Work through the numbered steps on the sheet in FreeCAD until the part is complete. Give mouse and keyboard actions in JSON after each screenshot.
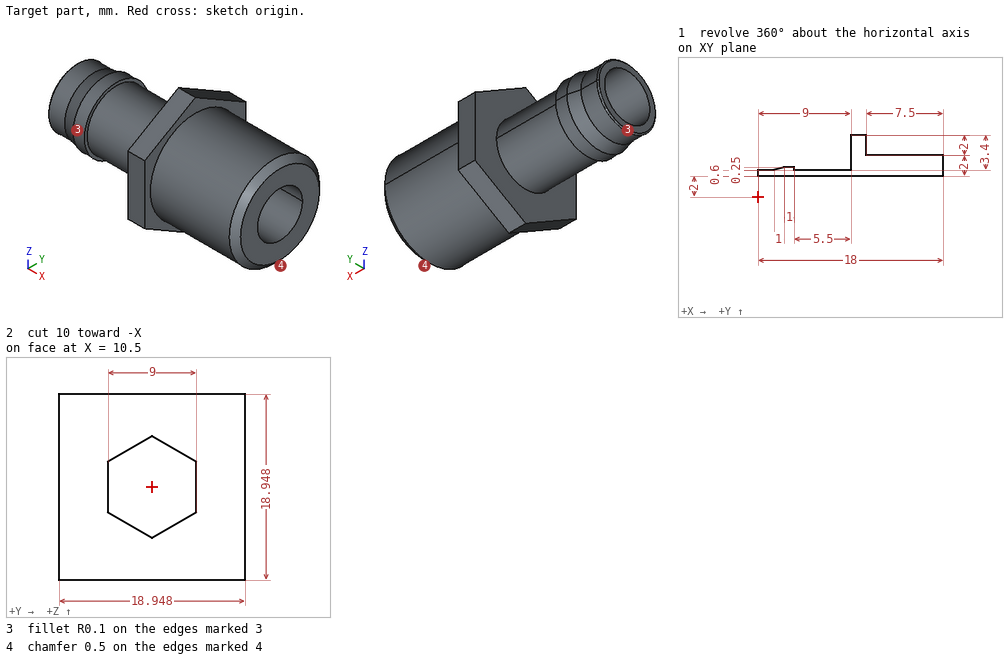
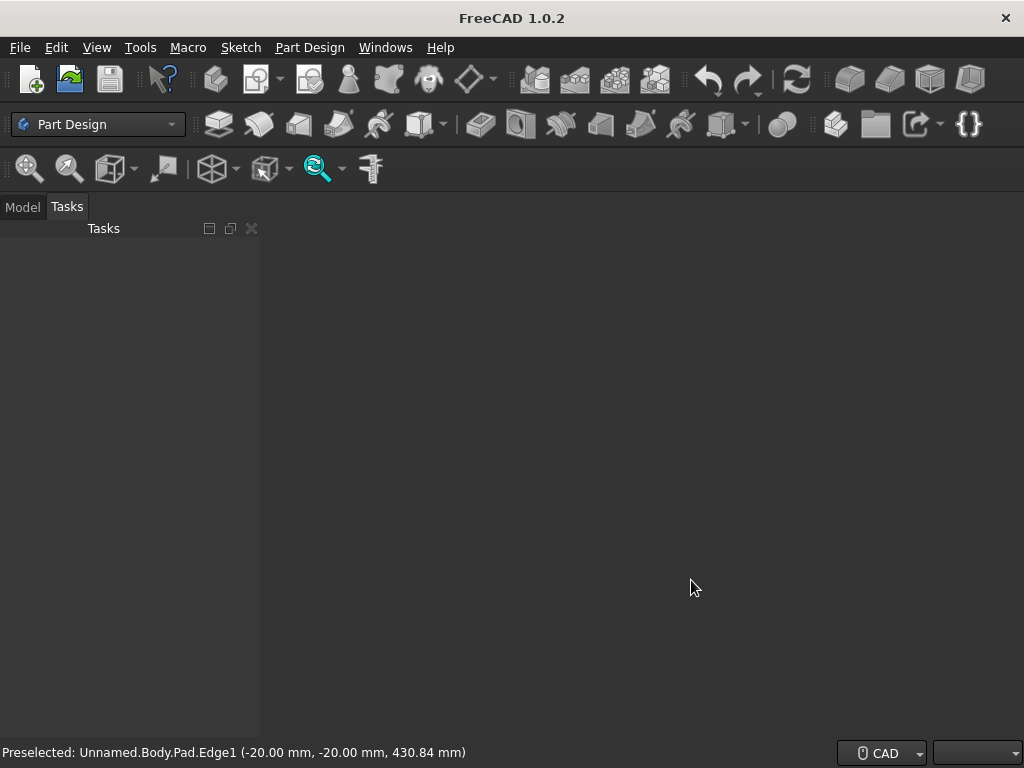
{"action": "left_click", "coordinate": [30, 80]}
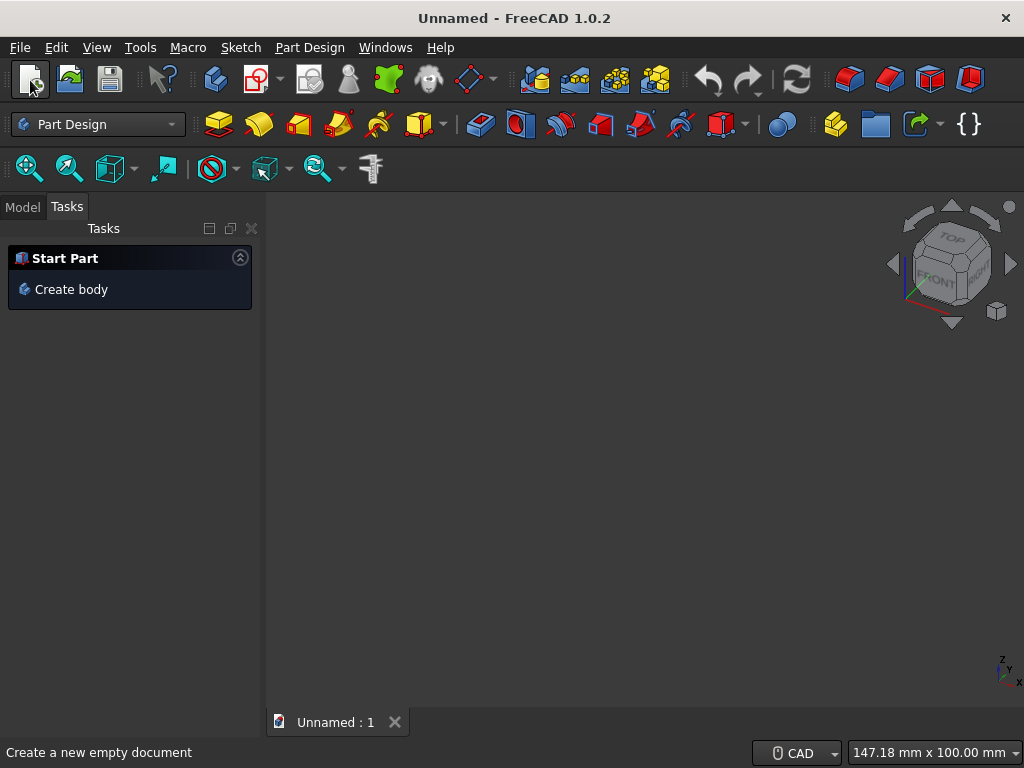
{"action": "left_click", "coordinate": [256, 80]}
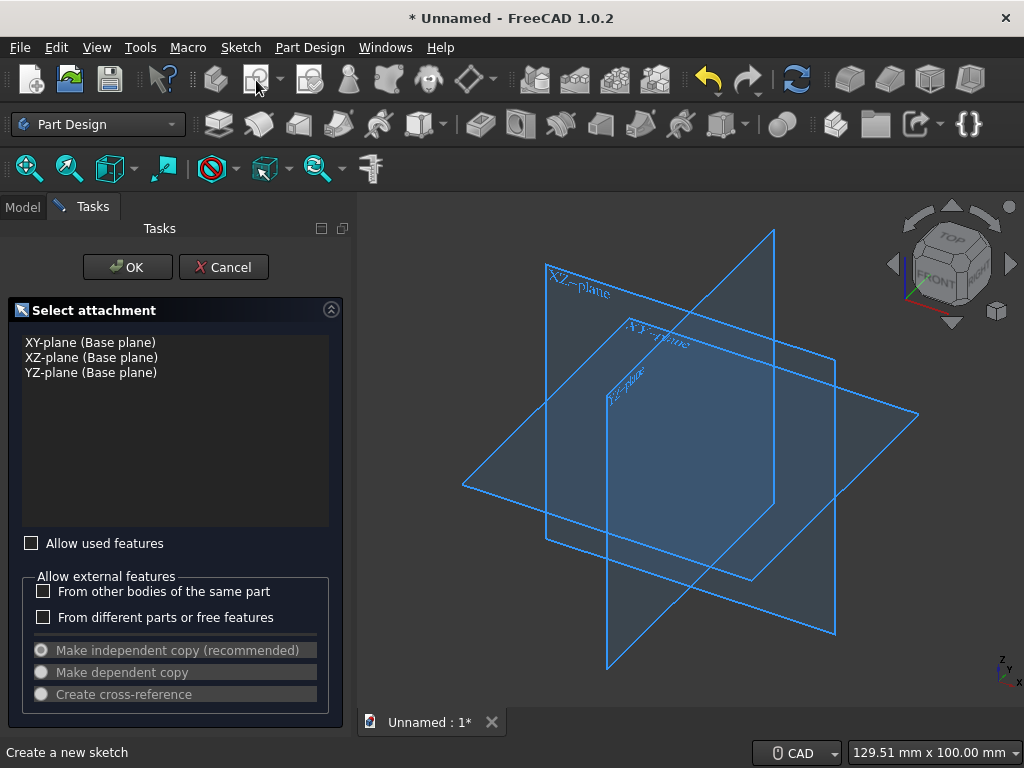
{"action": "left_click", "coordinate": [82, 342]}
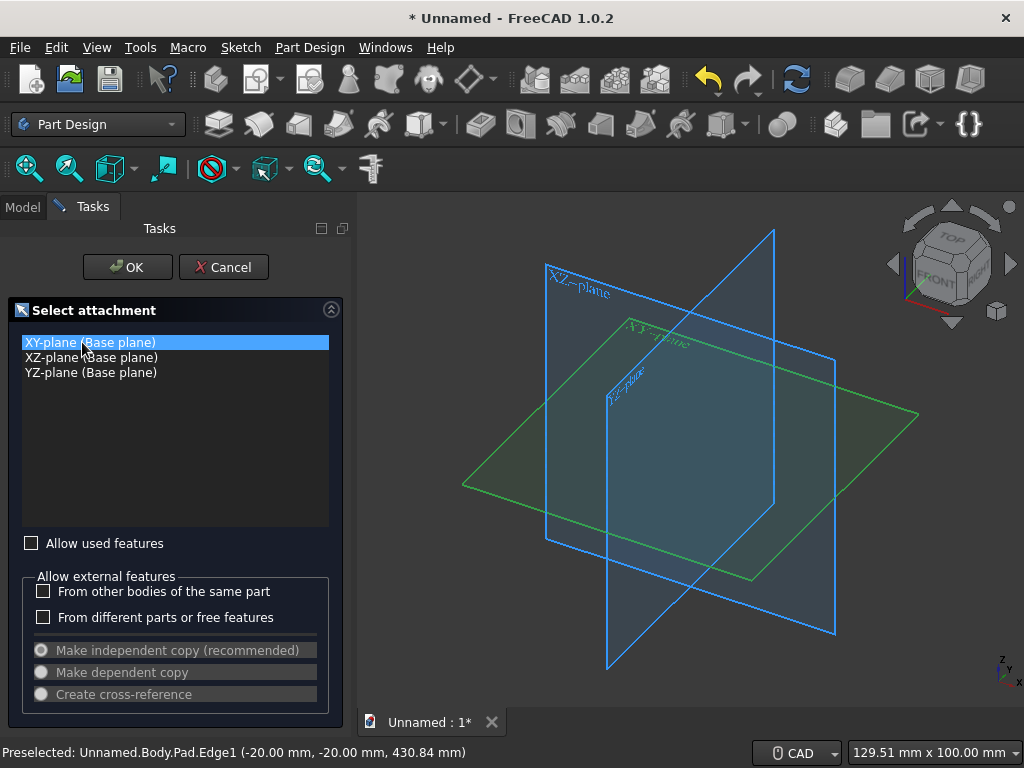
{"action": "left_click", "coordinate": [128, 267]}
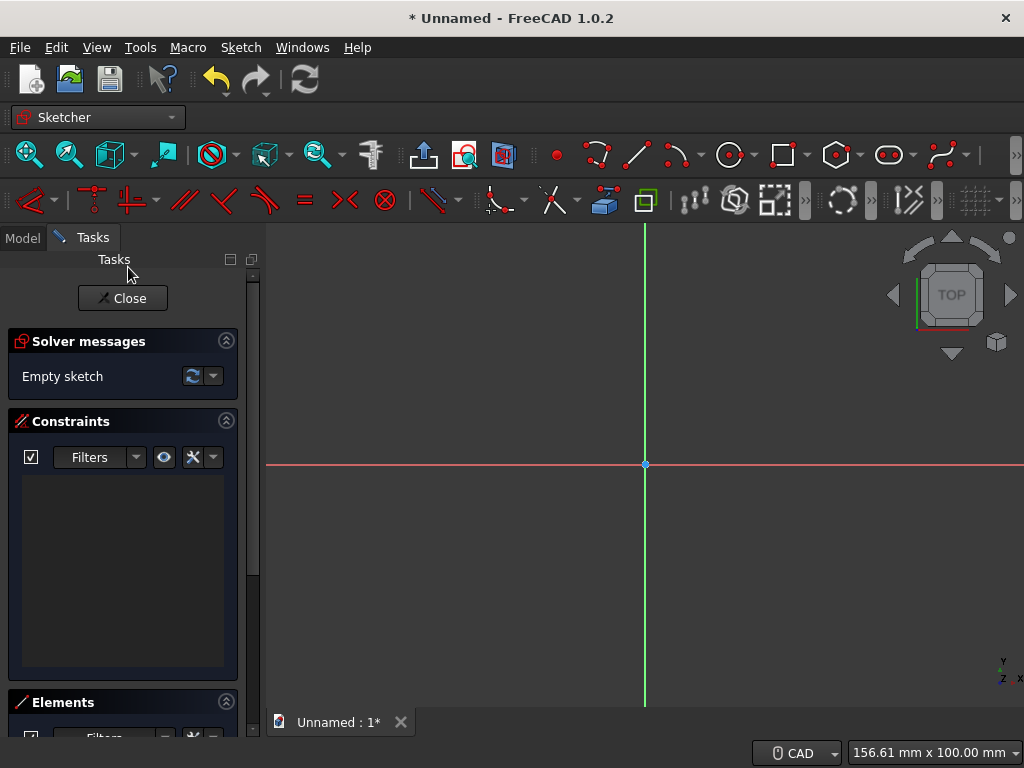
{"action": "scroll", "coordinate": [717, 447], "scroll_direction": "up", "scroll_amount": 8}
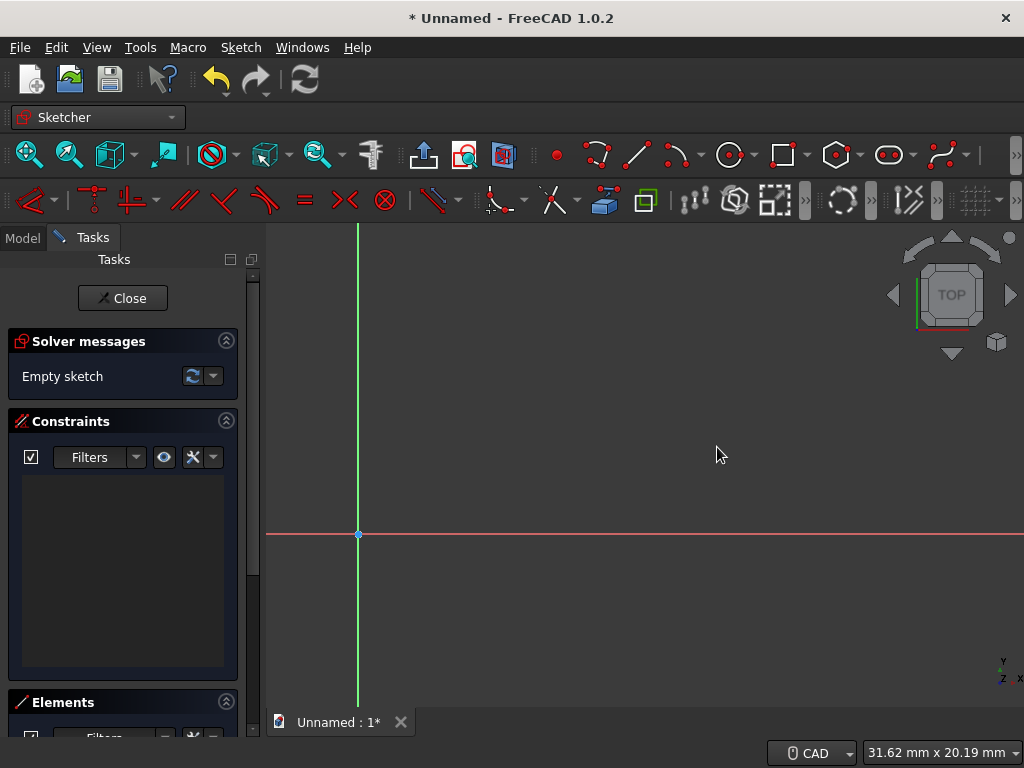
{"action": "left_click", "coordinate": [598, 156]}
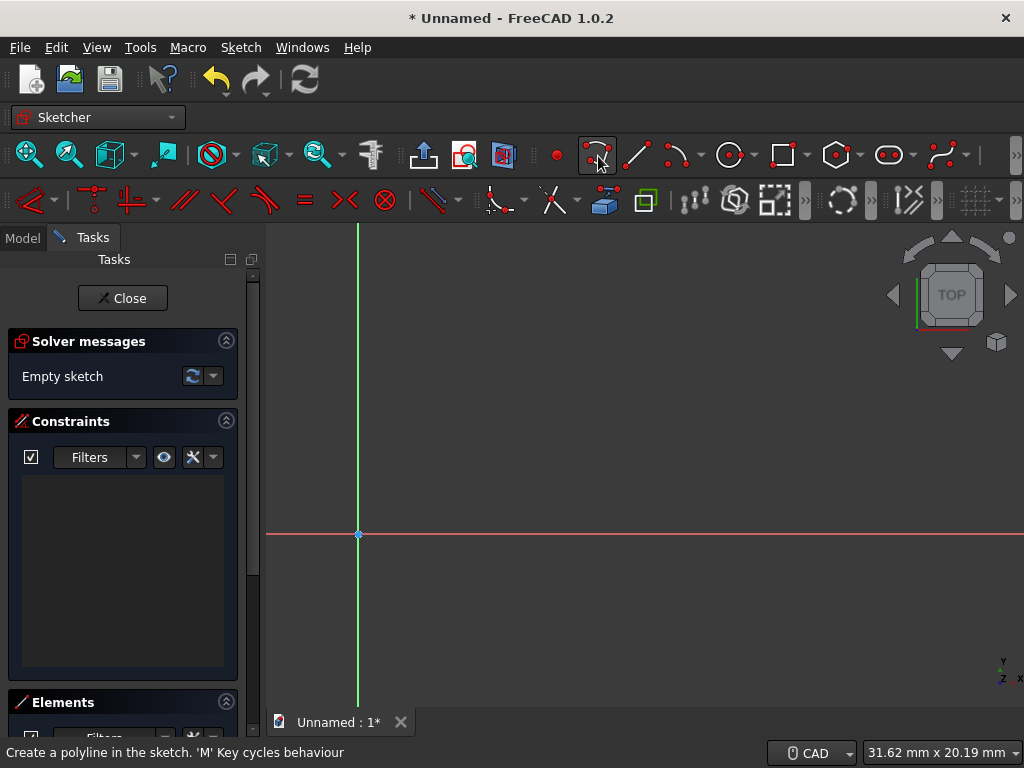
{"action": "left_click", "coordinate": [358, 486]}
{"action": "left_click", "coordinate": [790, 486]}
{"action": "left_click", "coordinate": [790, 438]}
{"action": "left_click", "coordinate": [610, 438]}
{"action": "left_click", "coordinate": [610, 390]}
{"action": "left_click", "coordinate": [574, 390]}
{"action": "left_click", "coordinate": [574, 472]}
{"action": "left_click", "coordinate": [442, 472]}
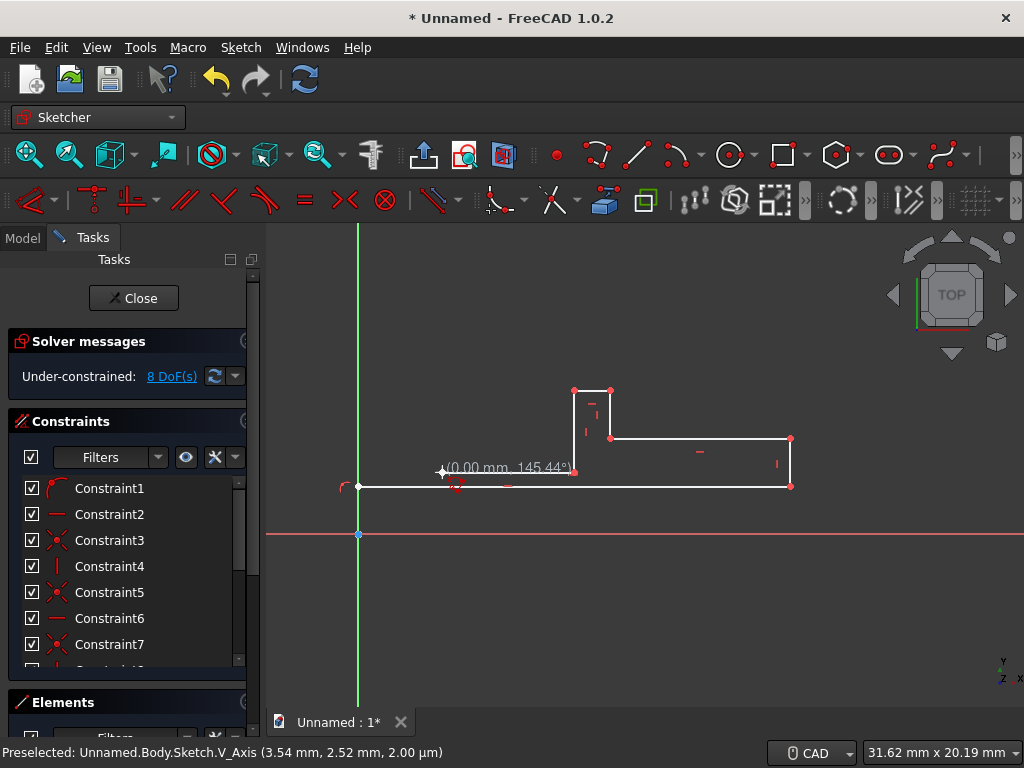
{"action": "scroll", "coordinate": [442, 466], "scroll_direction": "up", "scroll_amount": 5}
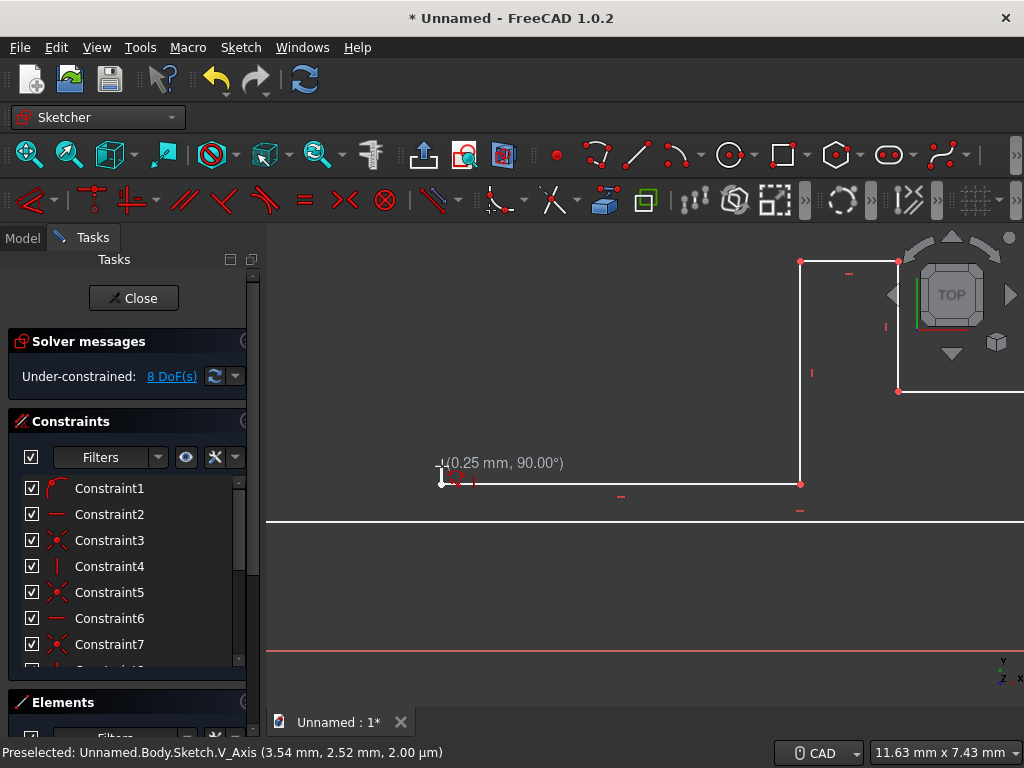
{"action": "left_click", "coordinate": [442, 465]}
{"action": "left_click", "coordinate": [376, 465]}
{"action": "left_click", "coordinate": [311, 481]}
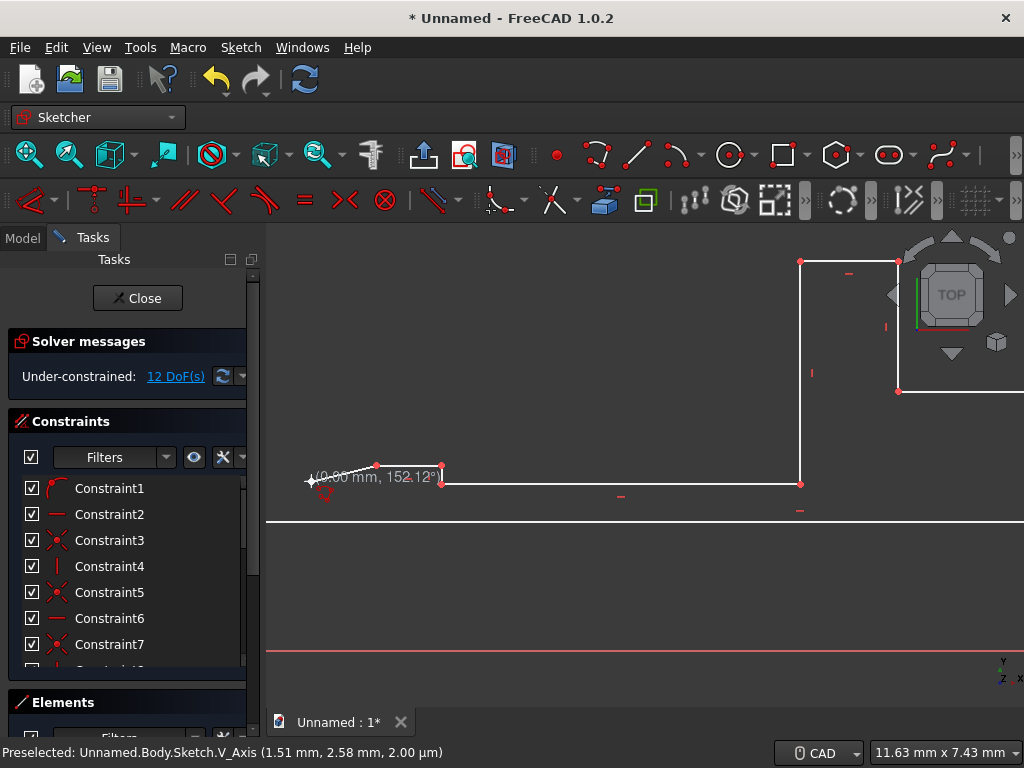
{"action": "scroll", "coordinate": [447, 471], "scroll_direction": "down", "scroll_amount": 5}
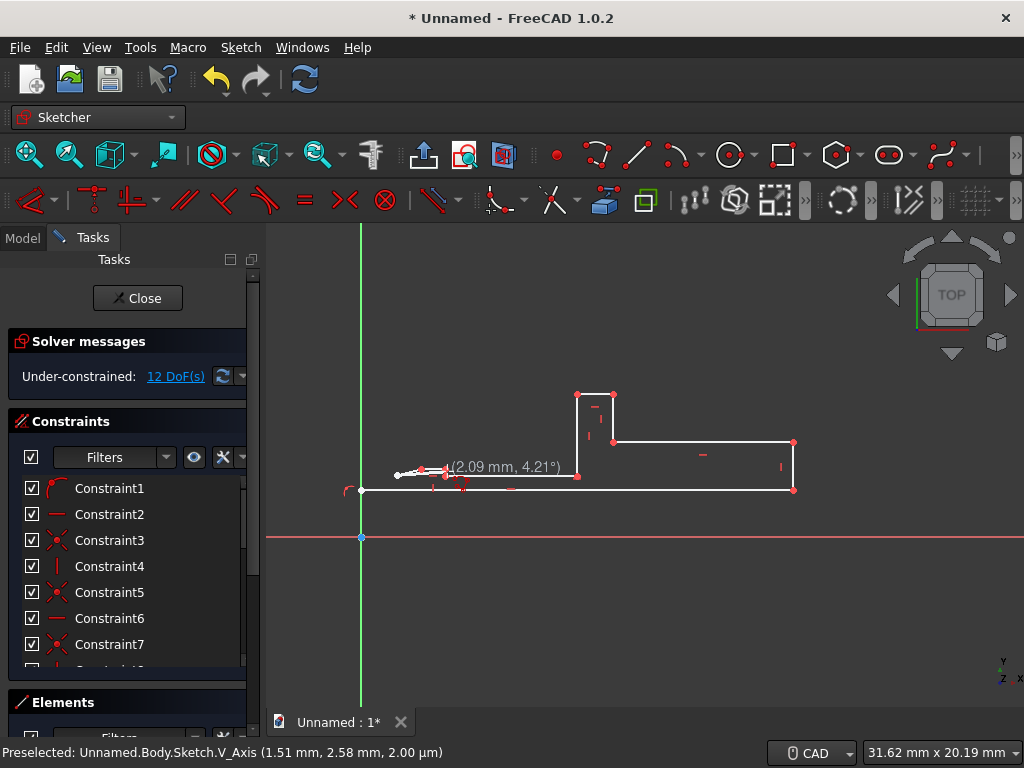
{"action": "left_click", "coordinate": [370, 475]}
{"action": "left_click", "coordinate": [361, 490]}
{"action": "key", "text": "Escape"}
{"action": "key", "text": "Escape"}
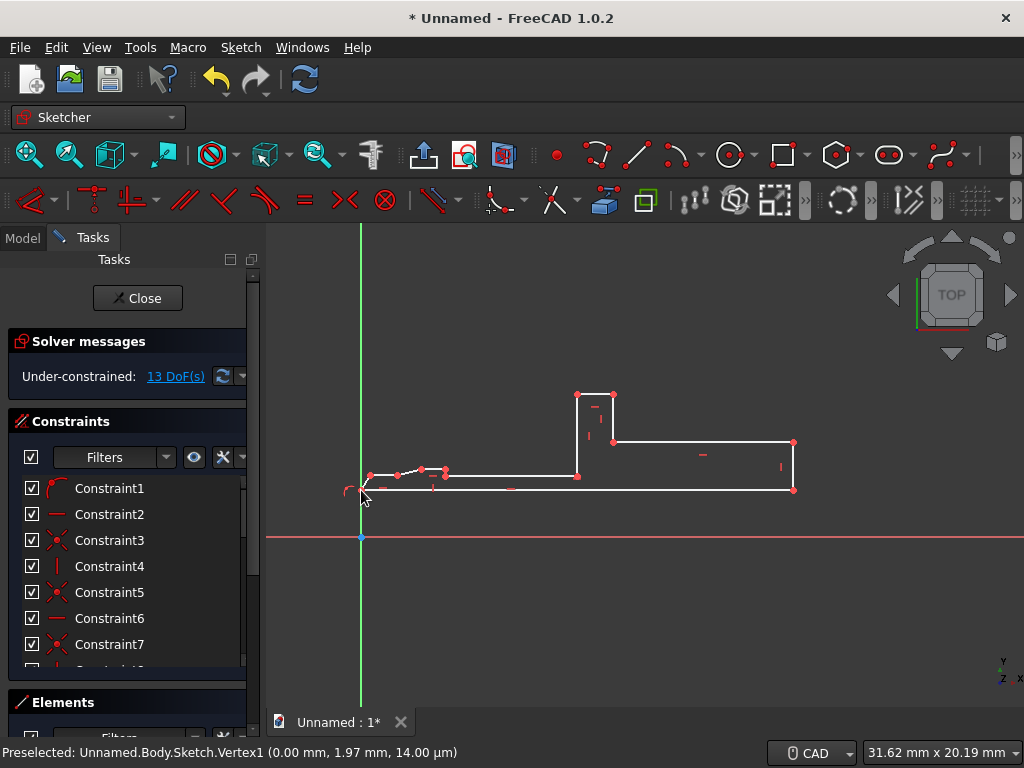
{"action": "scroll", "coordinate": [365, 484], "scroll_direction": "up", "scroll_amount": 5}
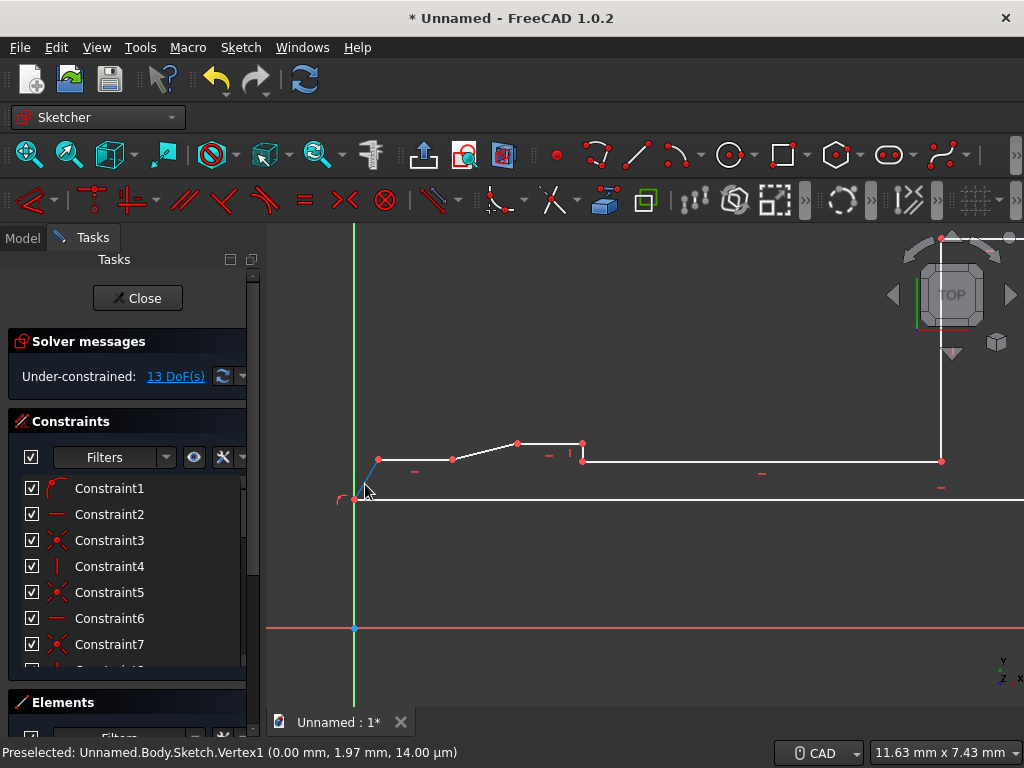
{"action": "left_click", "coordinate": [364, 484]}